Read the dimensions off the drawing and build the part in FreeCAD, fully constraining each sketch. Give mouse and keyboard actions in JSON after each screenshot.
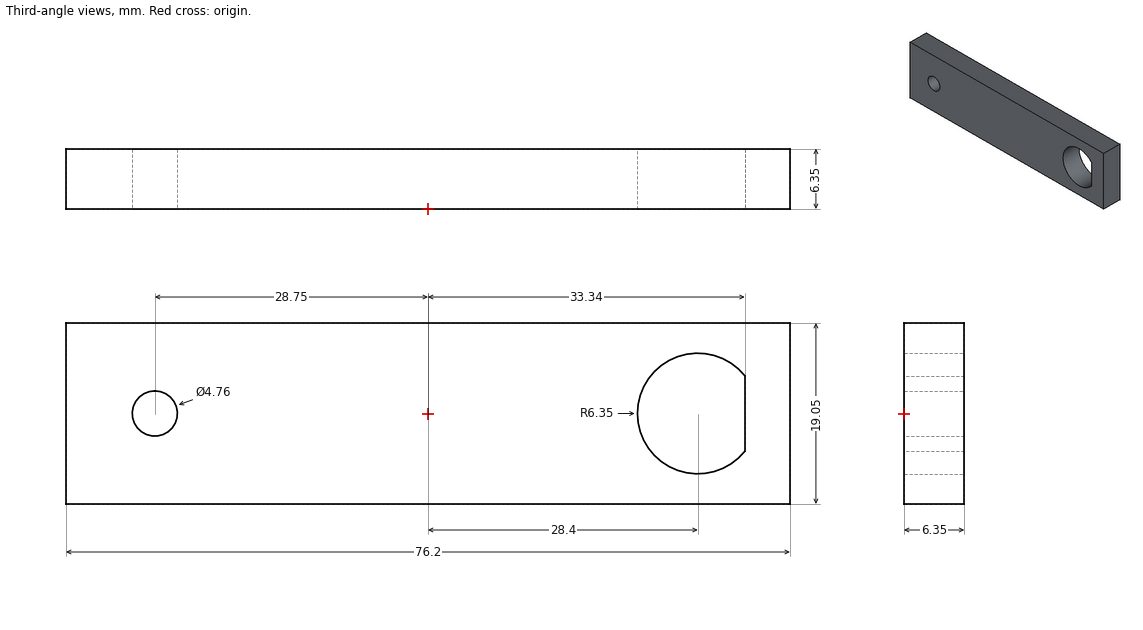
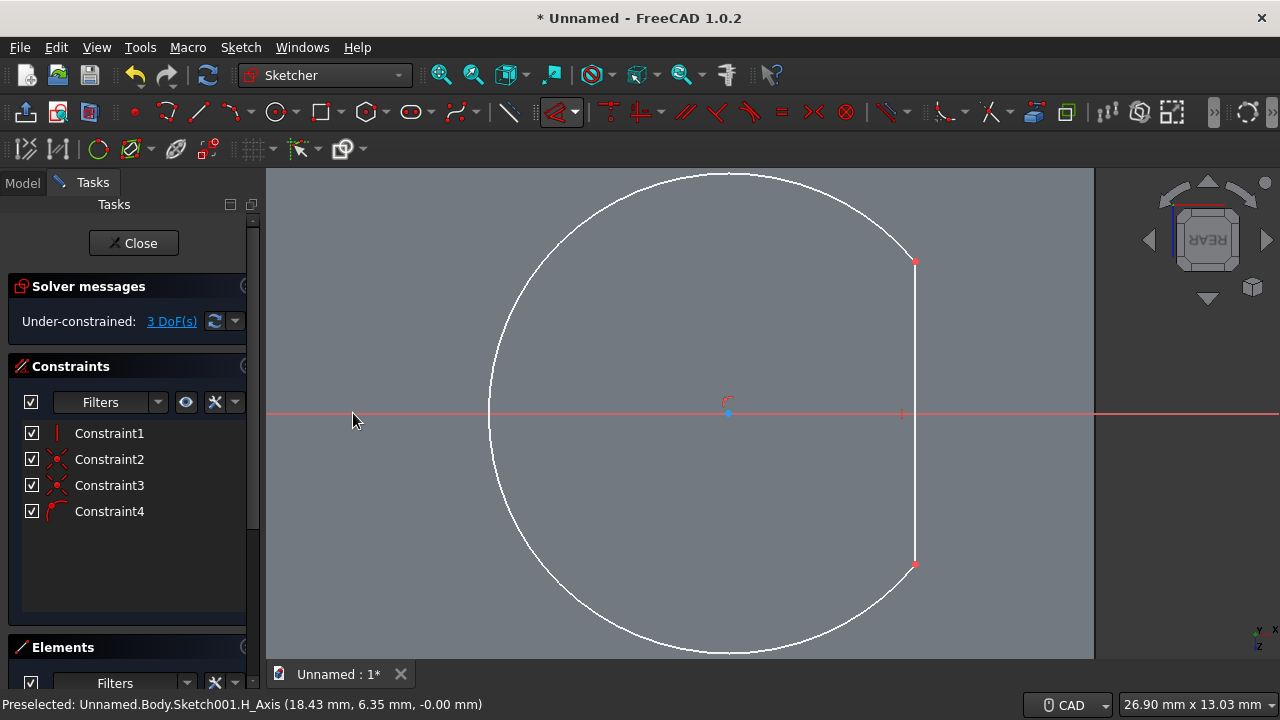
{"action": "left_click", "coordinate": [596, 214]}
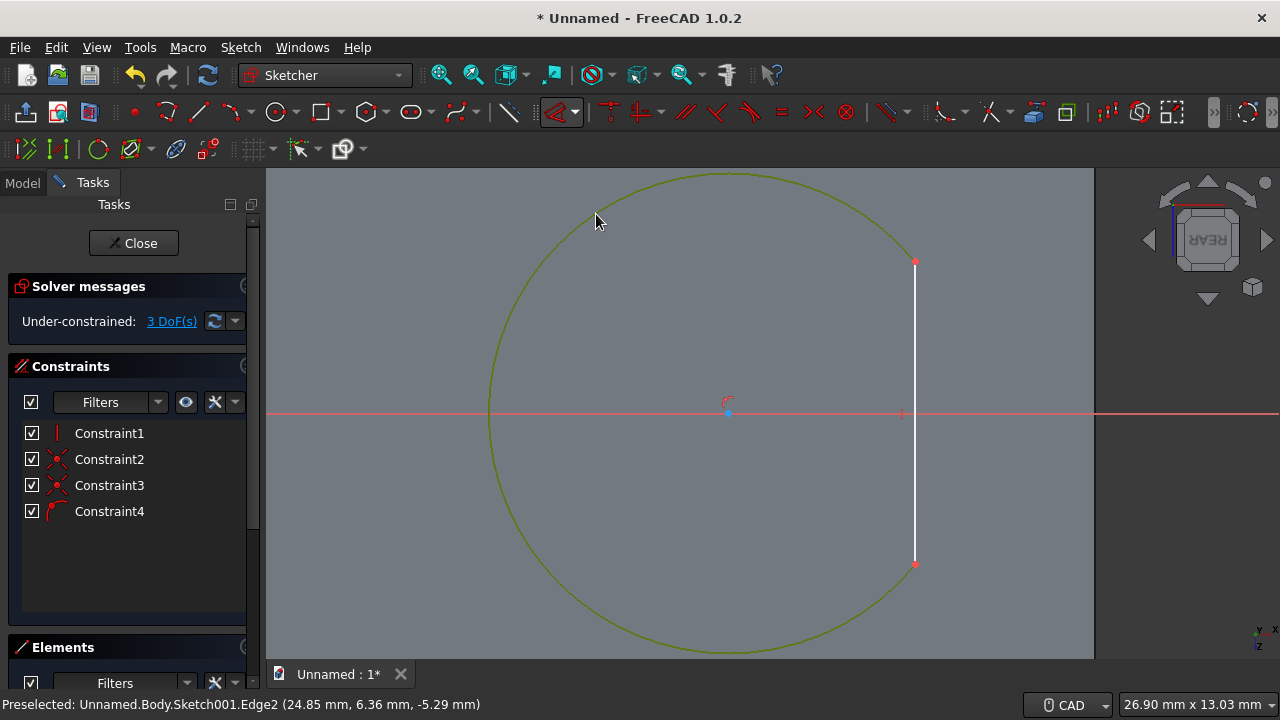
{"action": "key", "text": "k r"}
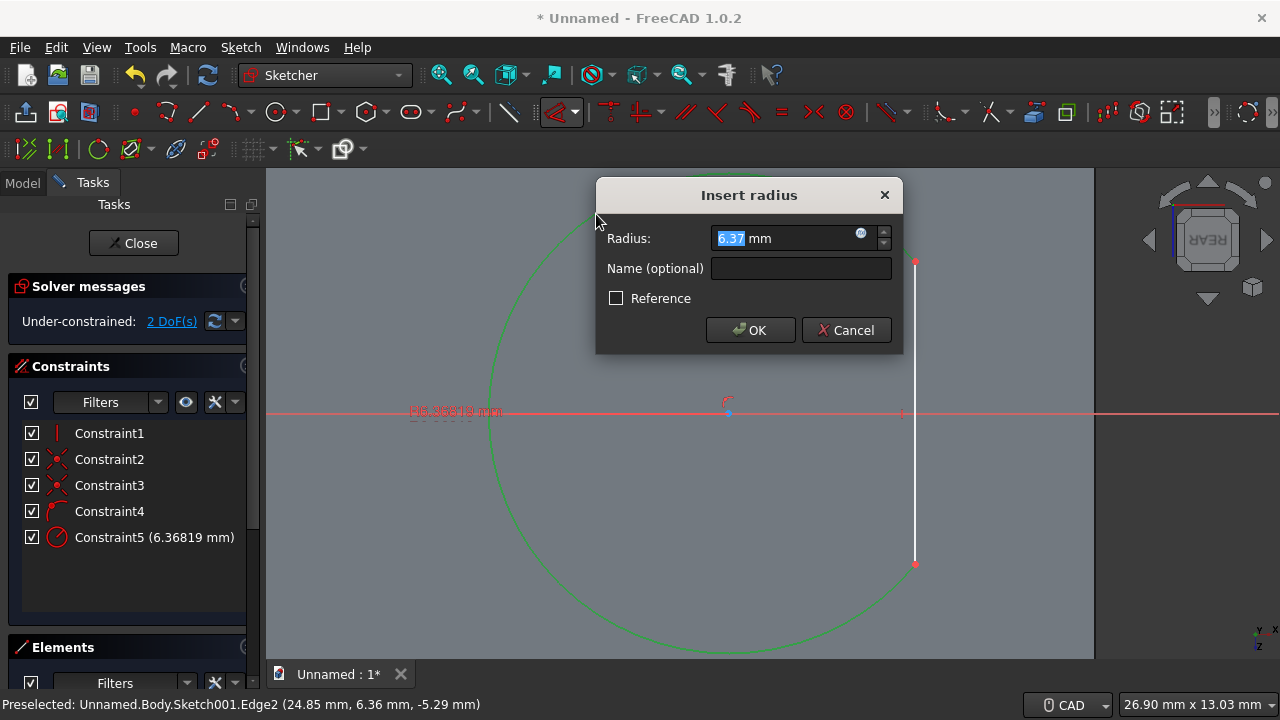
{"action": "type", "text": "6.35"}
{"action": "key", "text": "Return"}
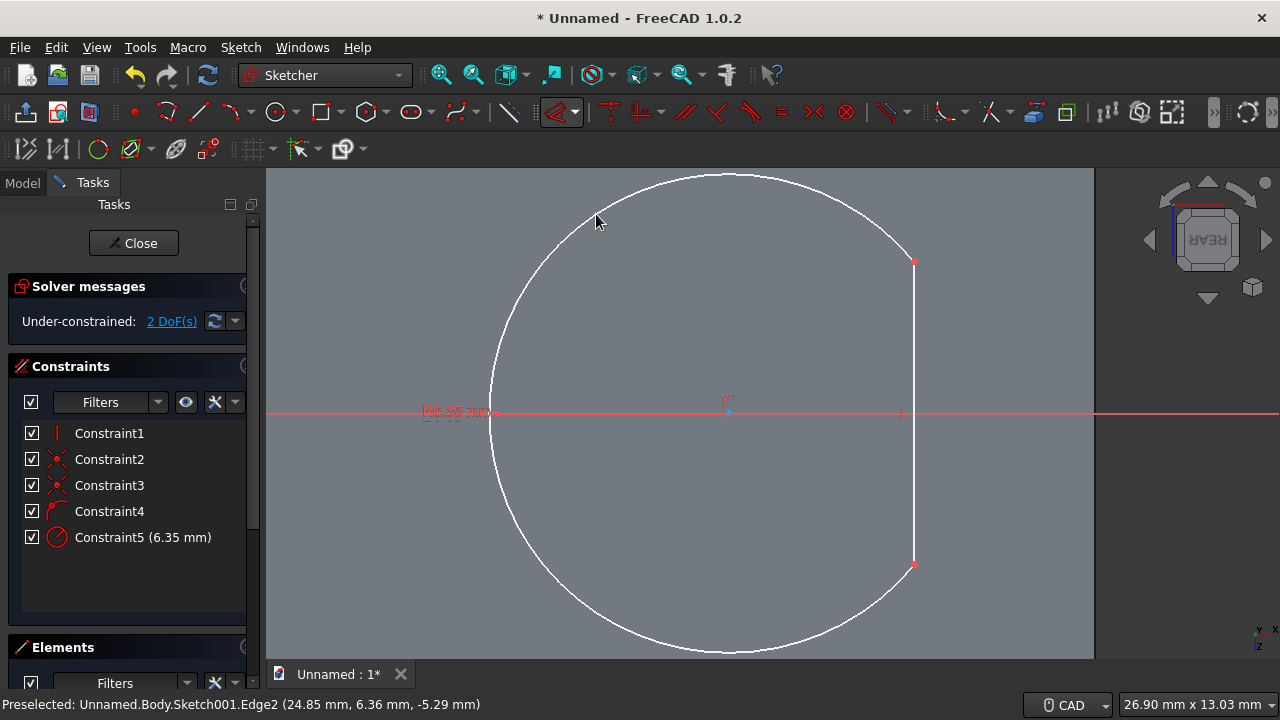
{"action": "left_click", "coordinate": [729, 413]}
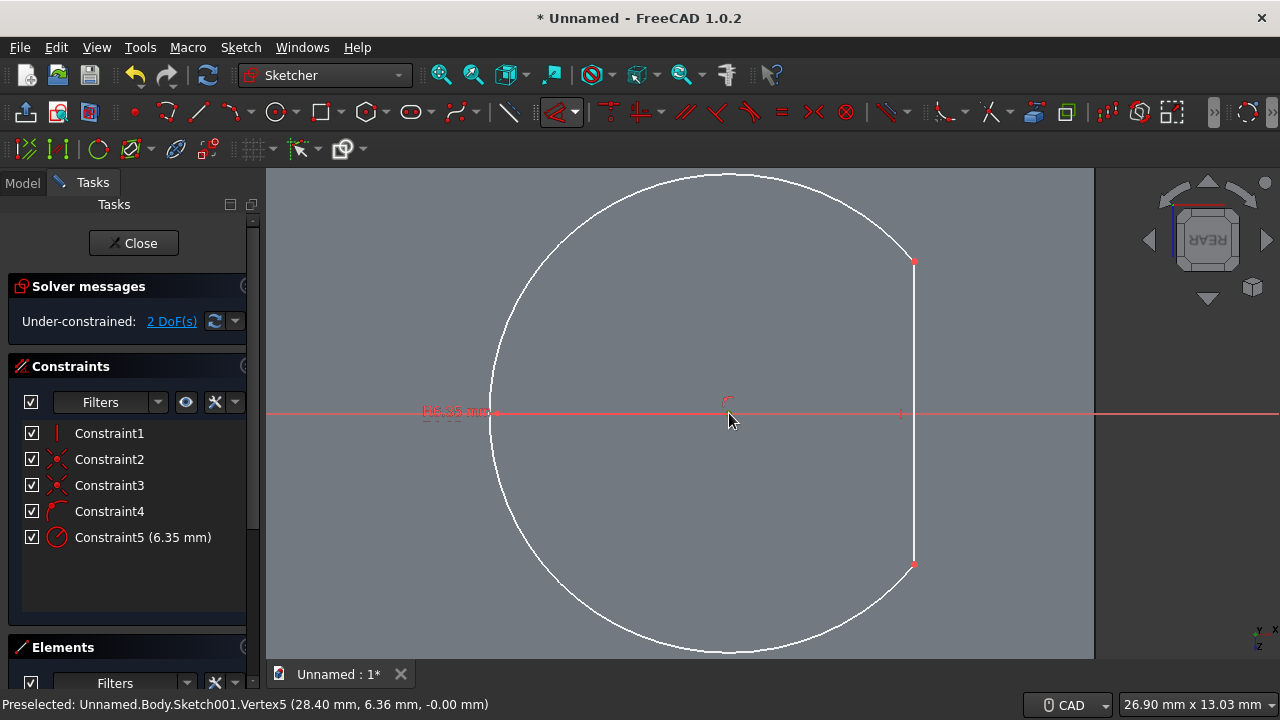
{"action": "key", "text": "l"}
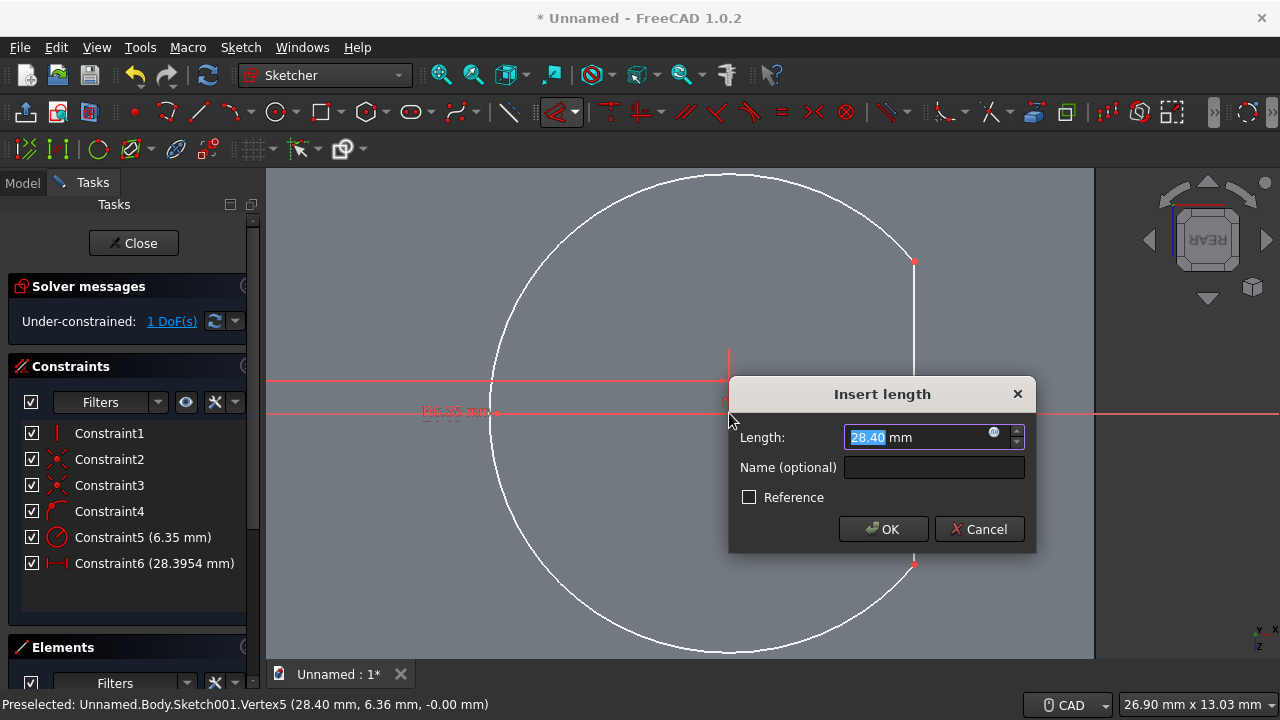
{"action": "type", "text": "28.4"}
{"action": "key", "text": "Return"}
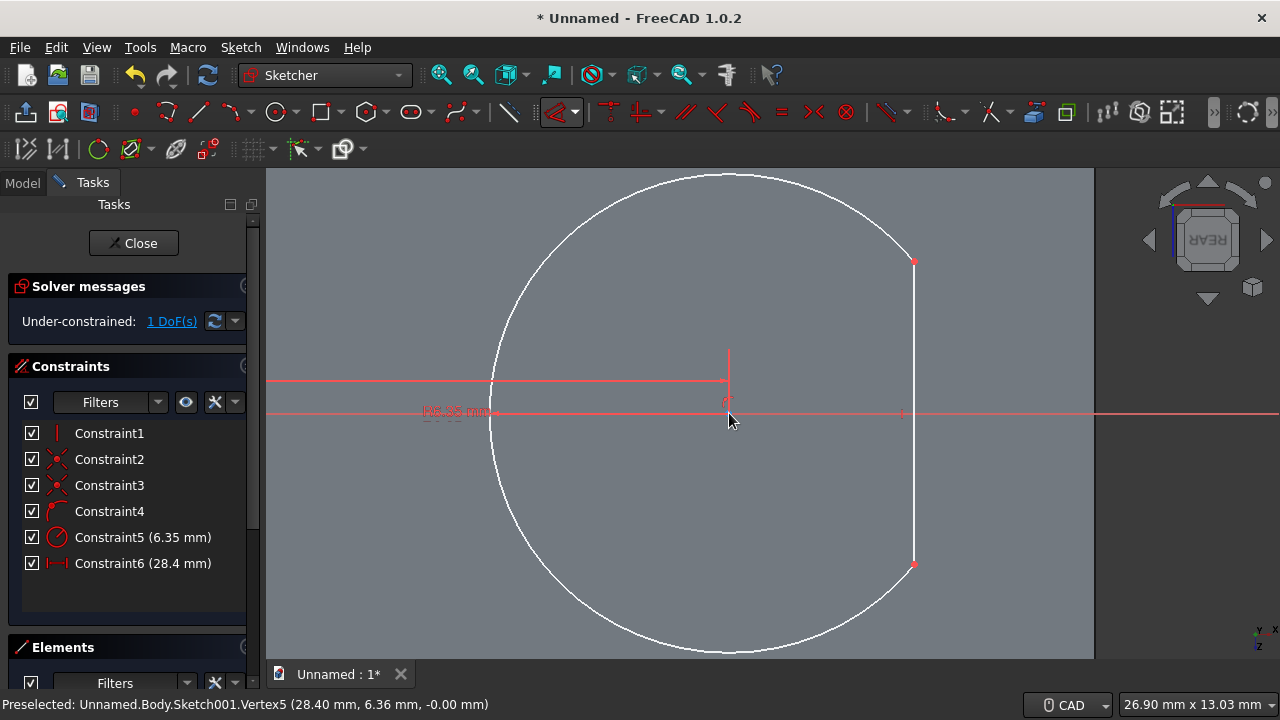
{"action": "left_click", "coordinate": [914, 565]}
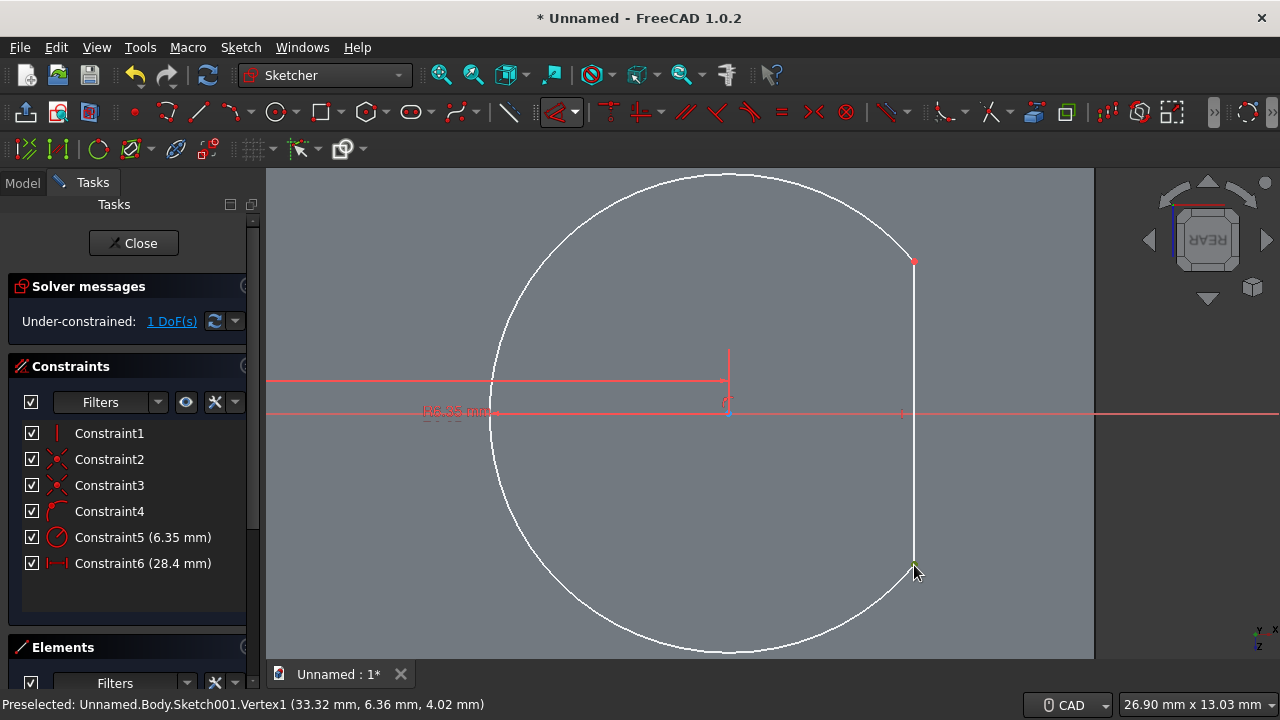
{"action": "key", "text": "l"}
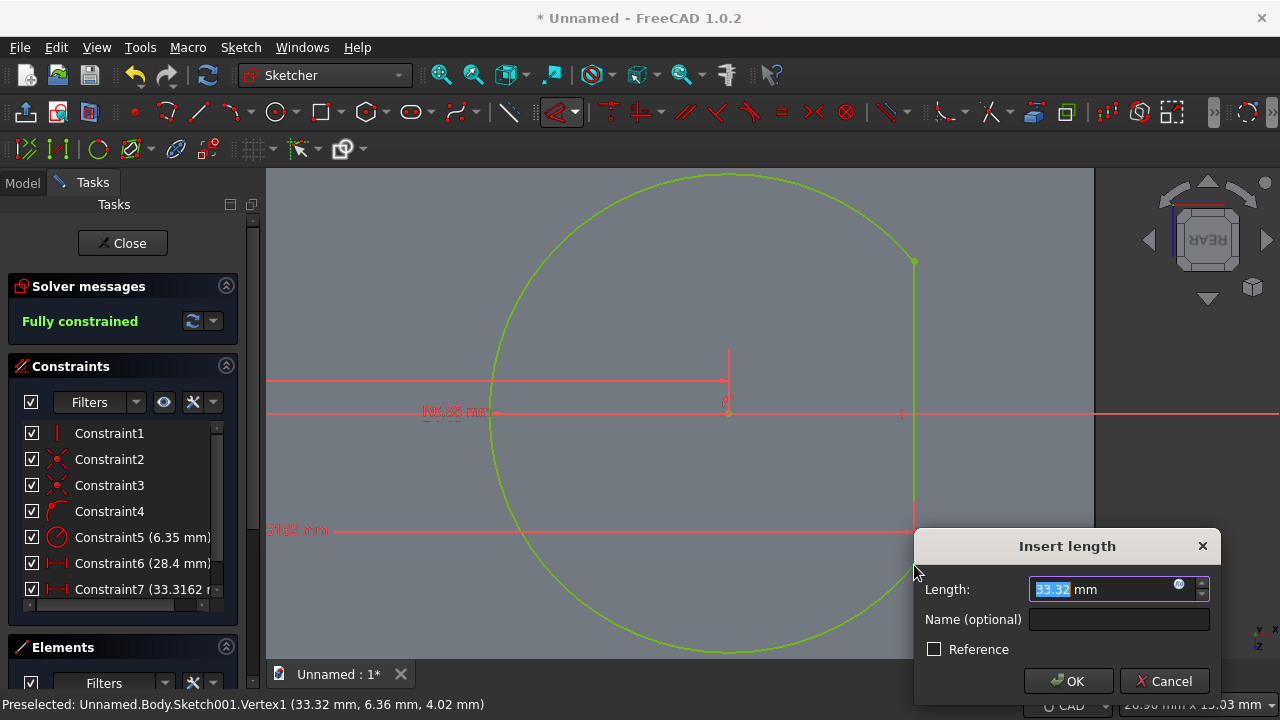
{"action": "type", "text": "33.34"}
{"action": "key", "text": "Return"}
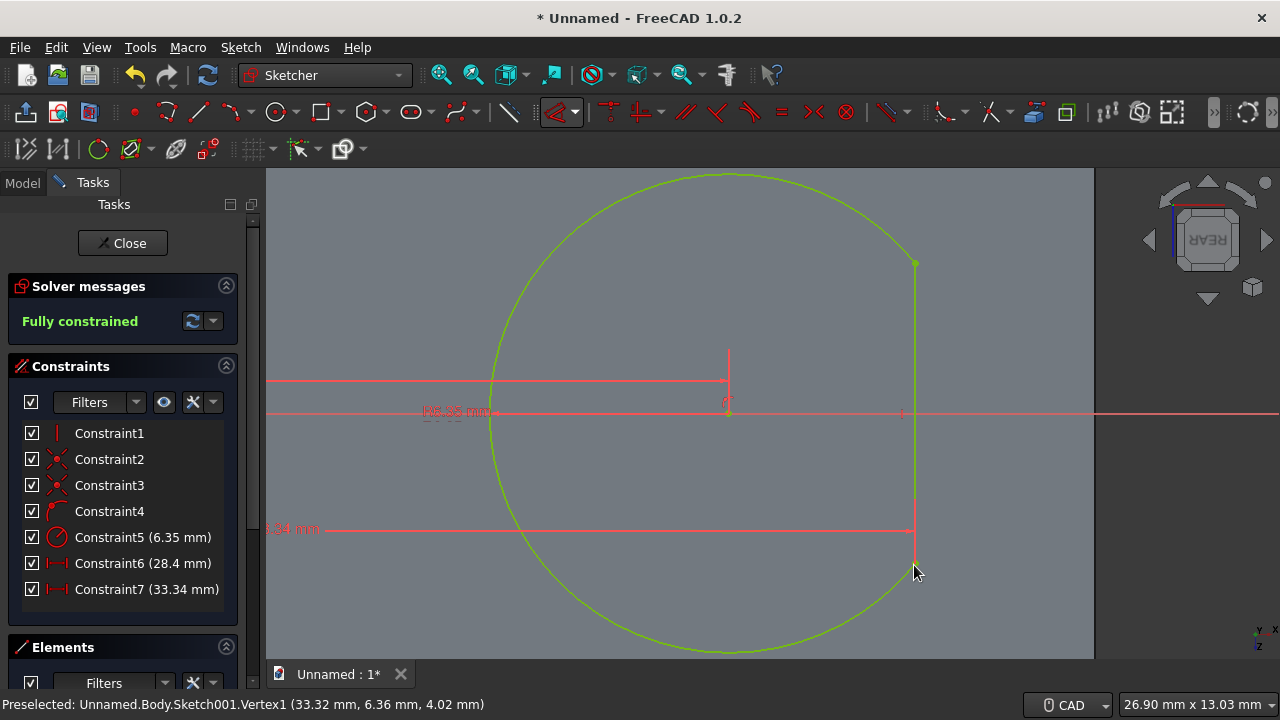
{"action": "left_click", "coordinate": [123, 243]}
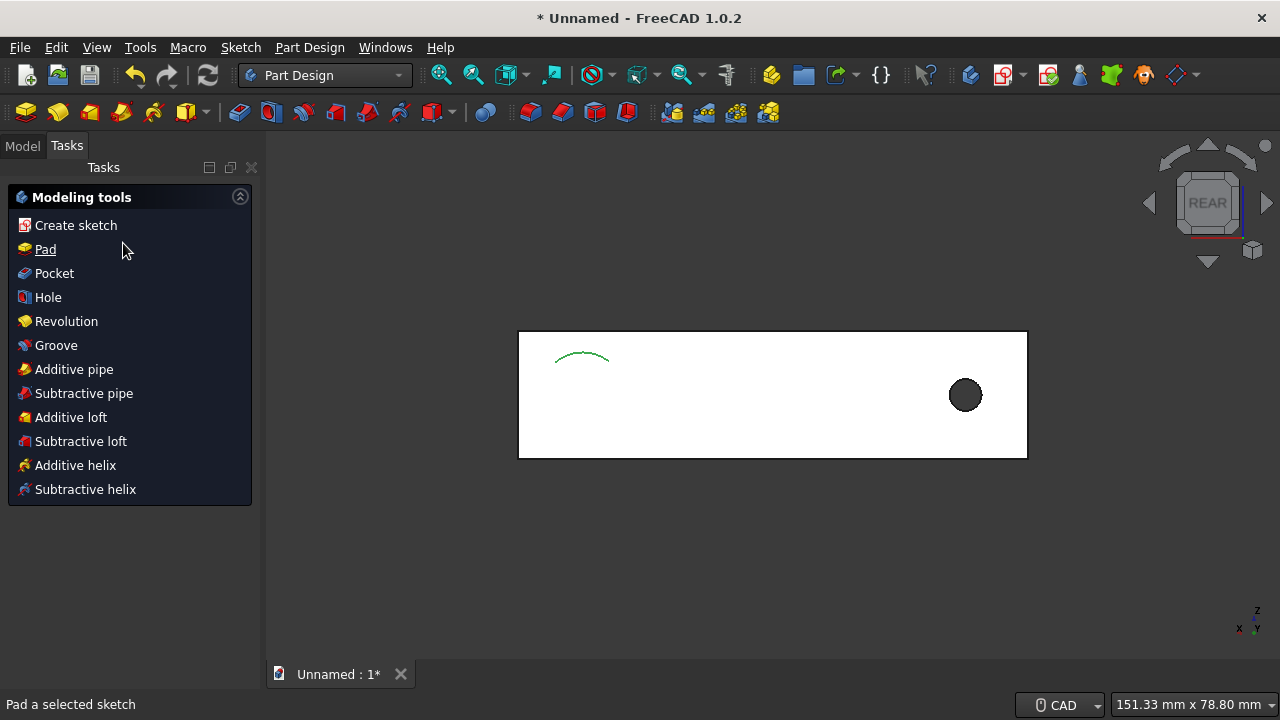
{"action": "left_click", "coordinate": [240, 112]}